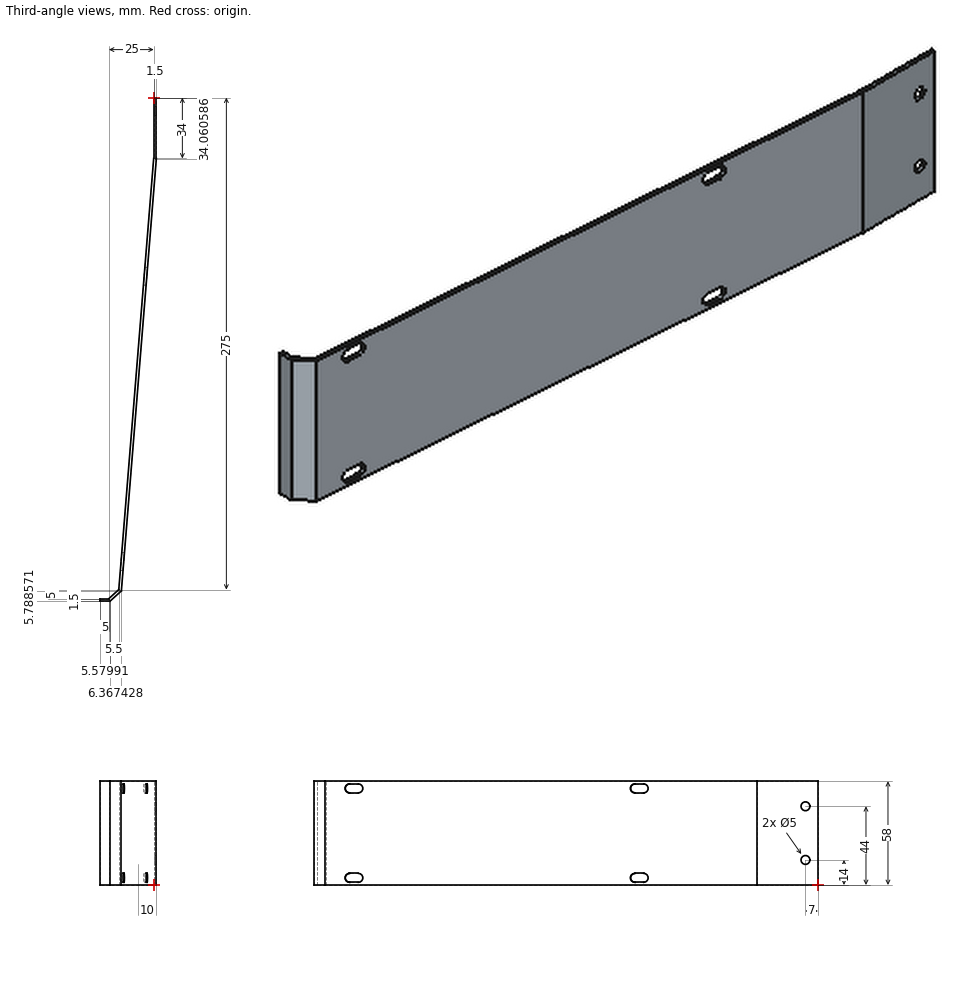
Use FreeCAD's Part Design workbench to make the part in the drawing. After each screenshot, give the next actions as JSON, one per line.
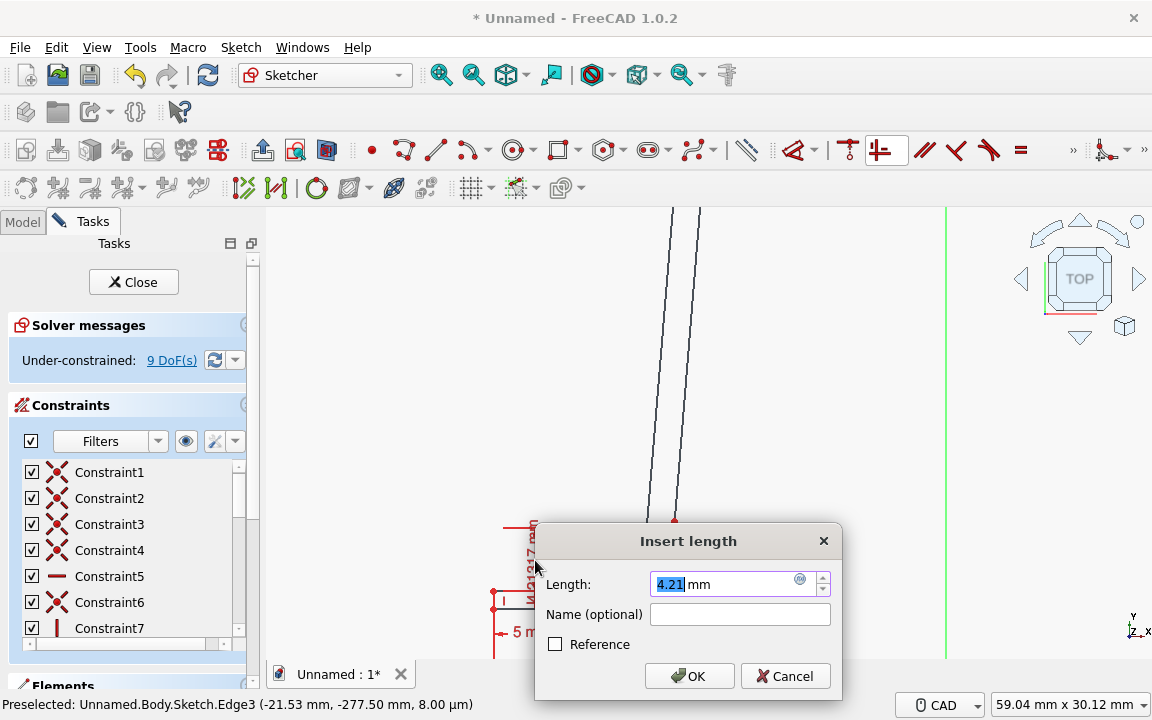
{"action": "type", "text": "5"}
{"action": "key", "text": "Return"}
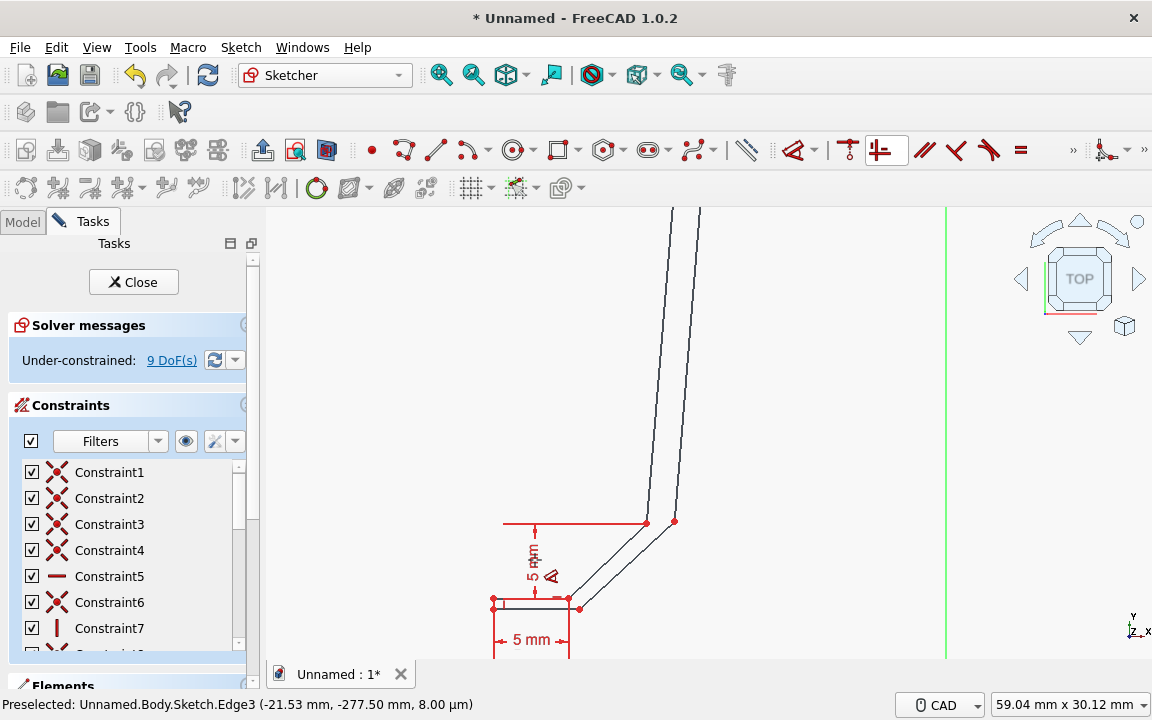
{"action": "scroll", "coordinate": [494, 604], "scroll_direction": "up", "scroll_amount": 3}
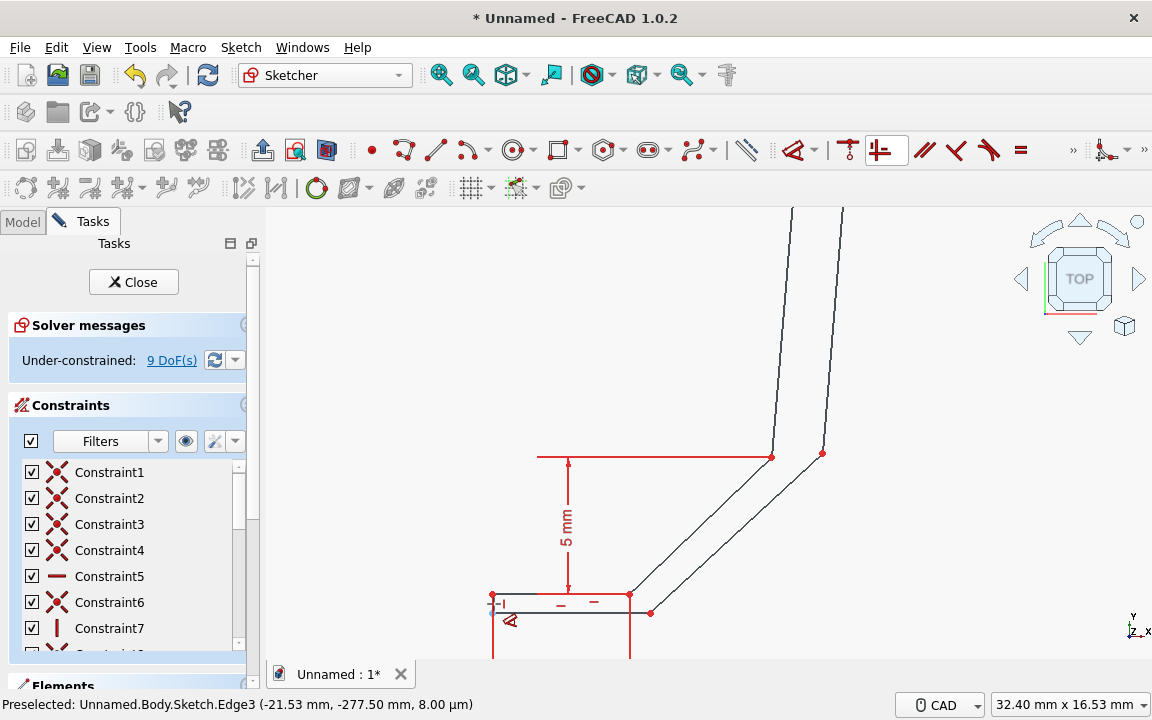
{"action": "left_click", "coordinate": [493, 604]}
{"action": "left_click", "coordinate": [459, 604]}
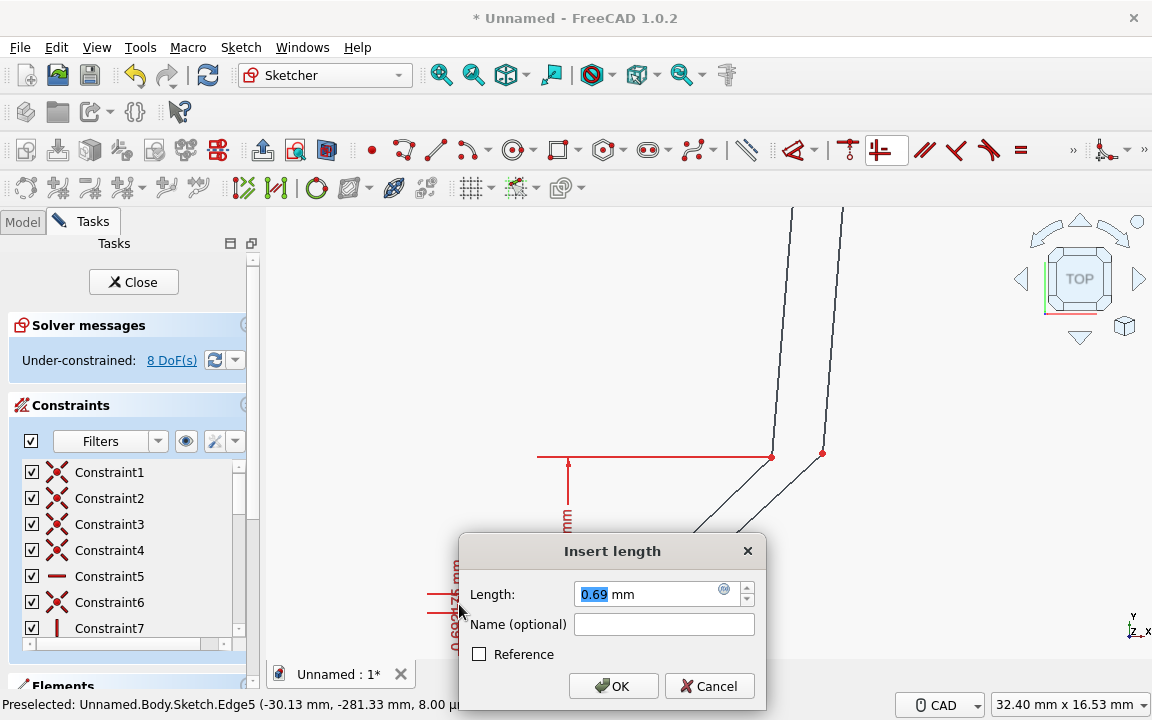
{"action": "type", "text": "1.5"}
{"action": "key", "text": "Return"}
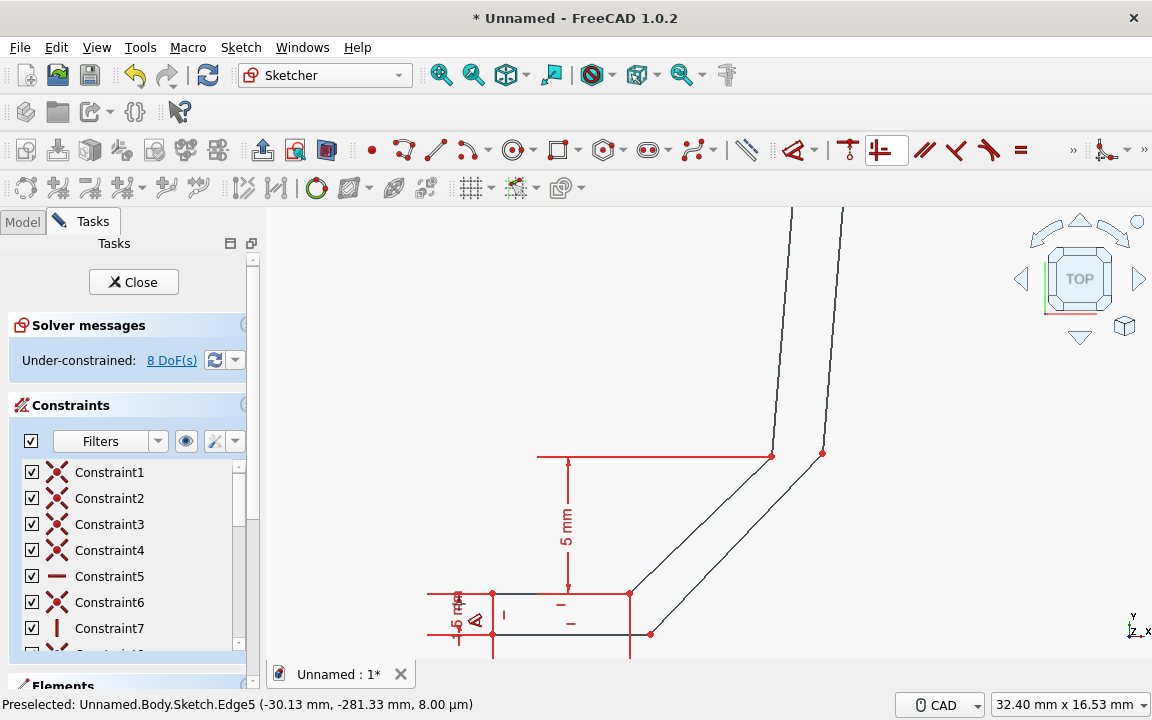
{"action": "scroll", "coordinate": [628, 589], "scroll_direction": "down", "scroll_amount": 16}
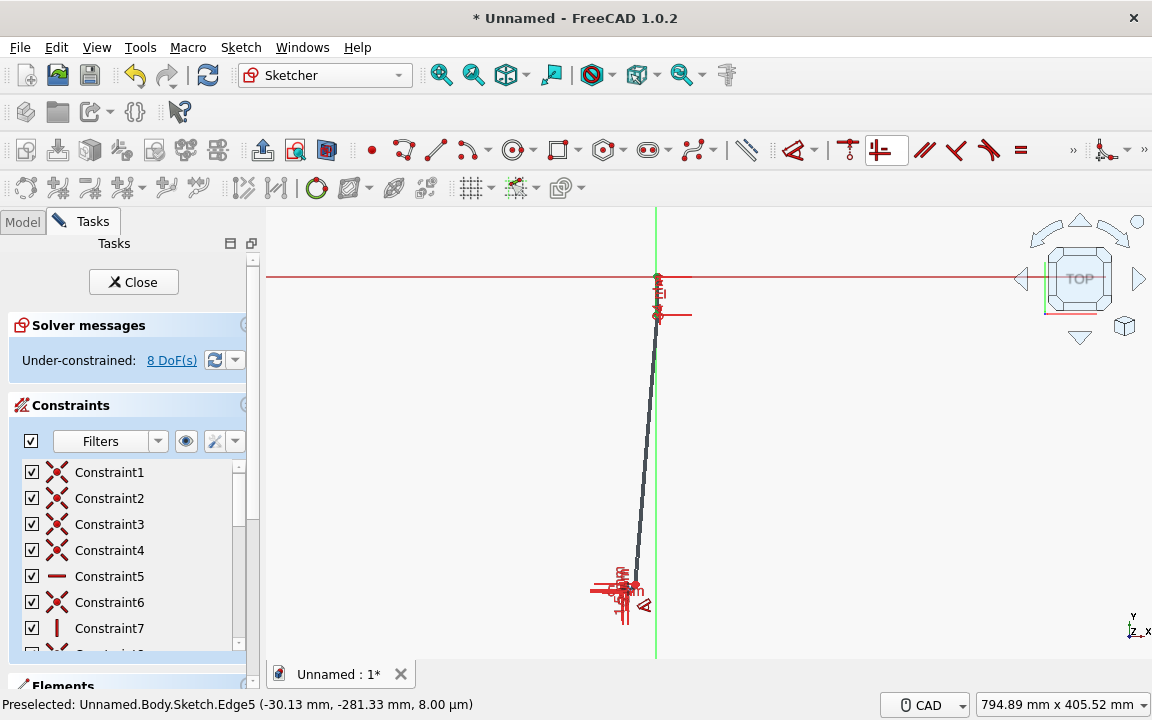
{"action": "scroll", "coordinate": [658, 277], "scroll_direction": "up", "scroll_amount": 16}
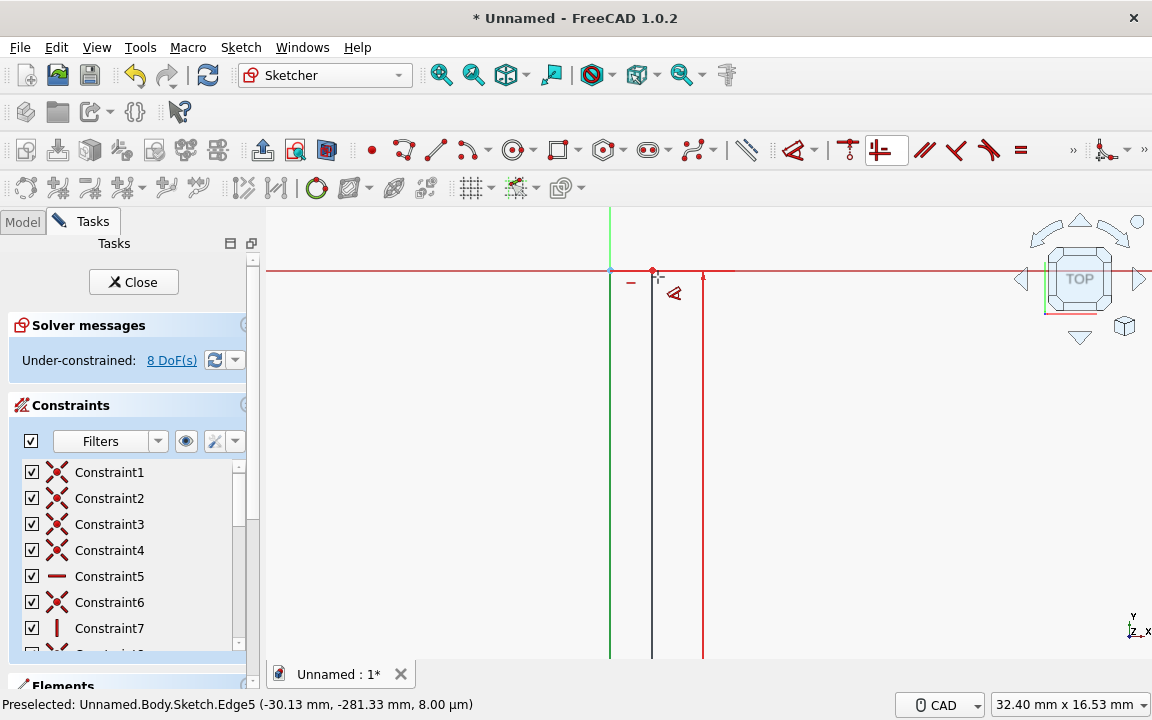
{"action": "left_click", "coordinate": [639, 271]}
{"action": "left_click", "coordinate": [631, 237]}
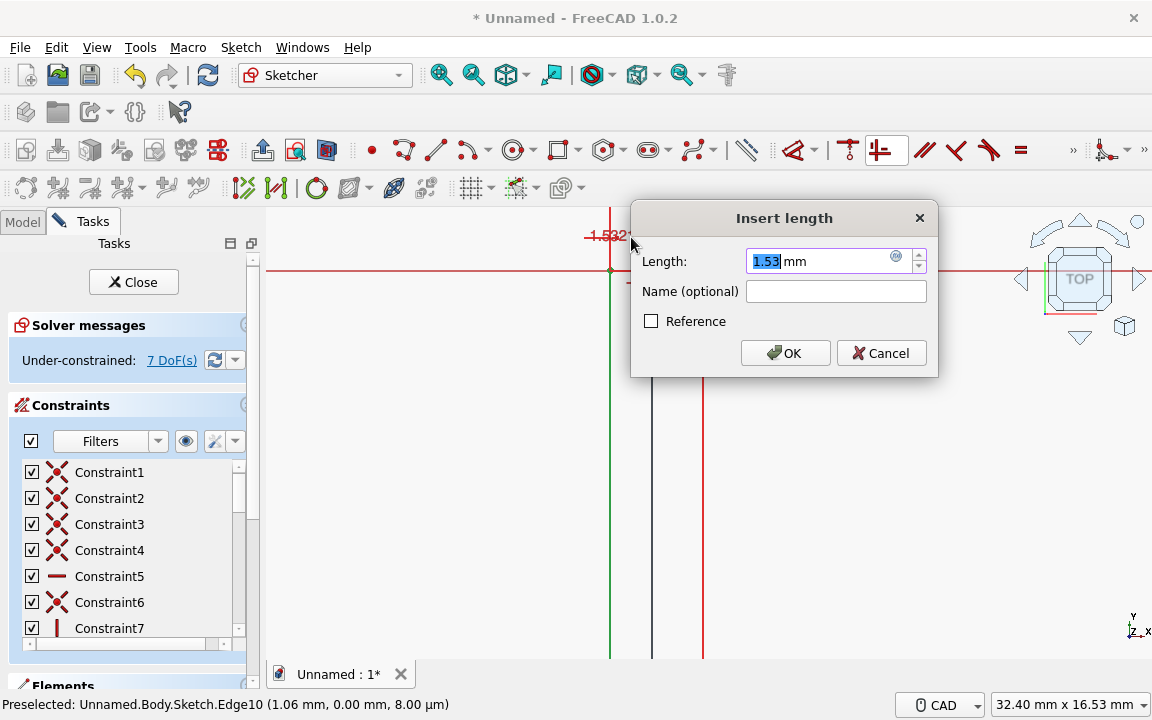
{"action": "type", "text": "1.5"}
{"action": "key", "text": "Return"}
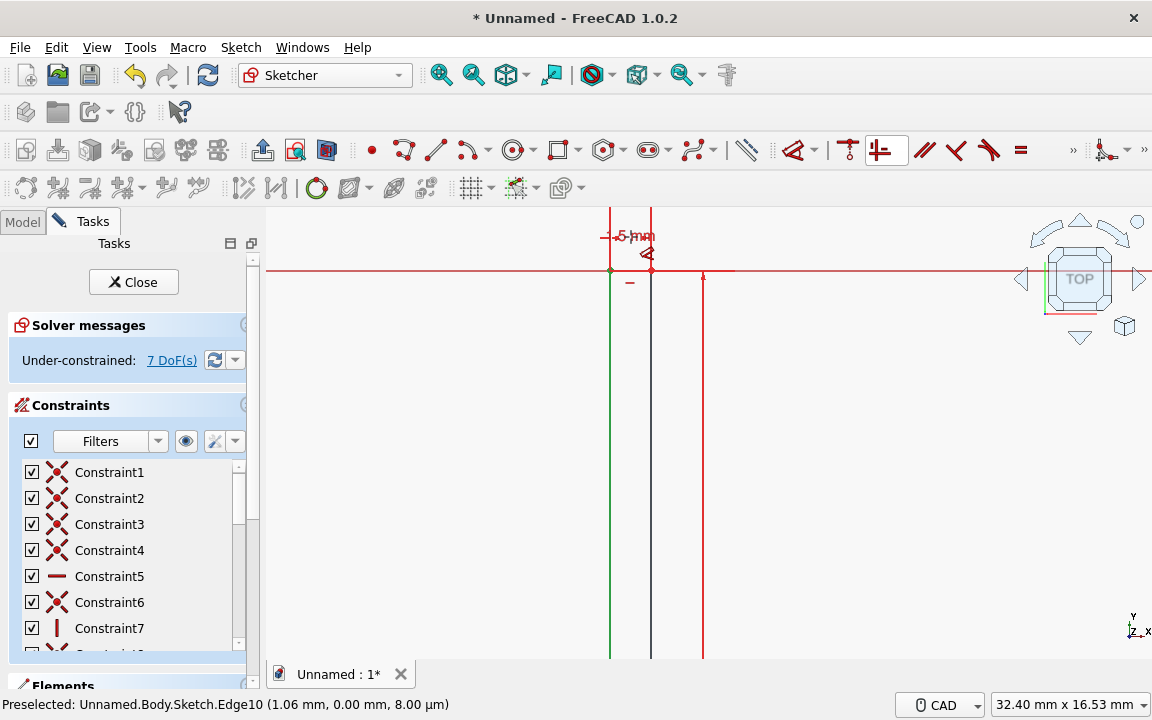
{"action": "scroll", "coordinate": [658, 276], "scroll_direction": "down", "scroll_amount": 16}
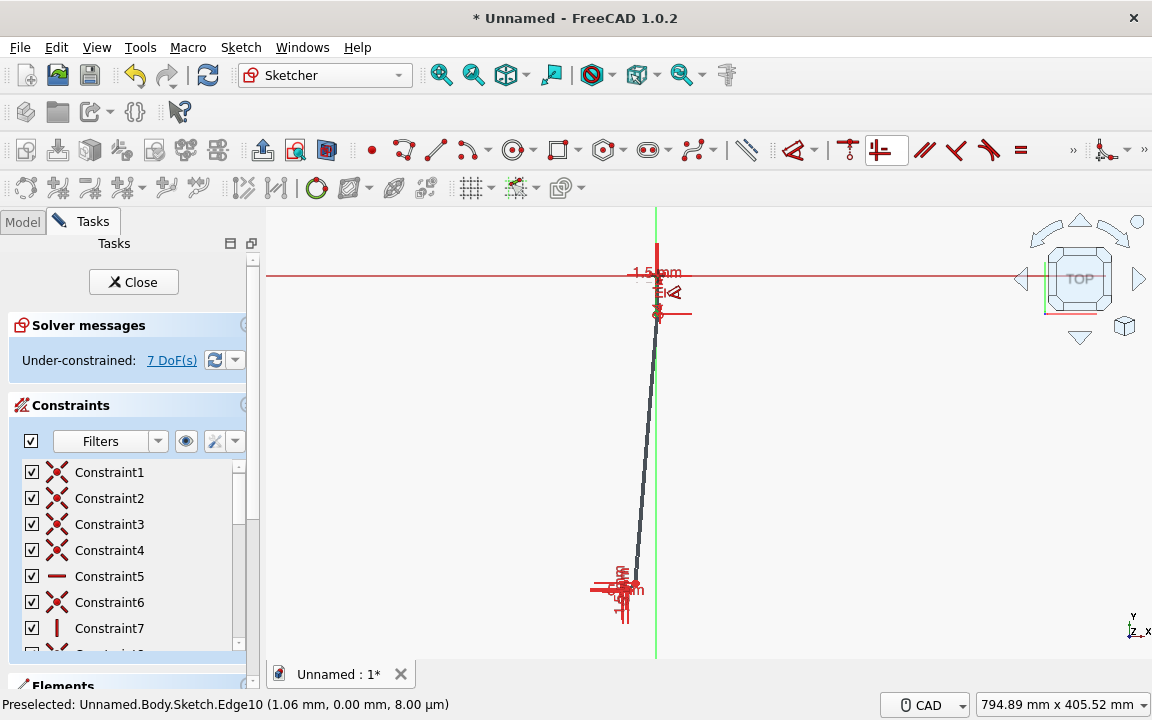
{"action": "scroll", "coordinate": [628, 589], "scroll_direction": "up", "scroll_amount": 10}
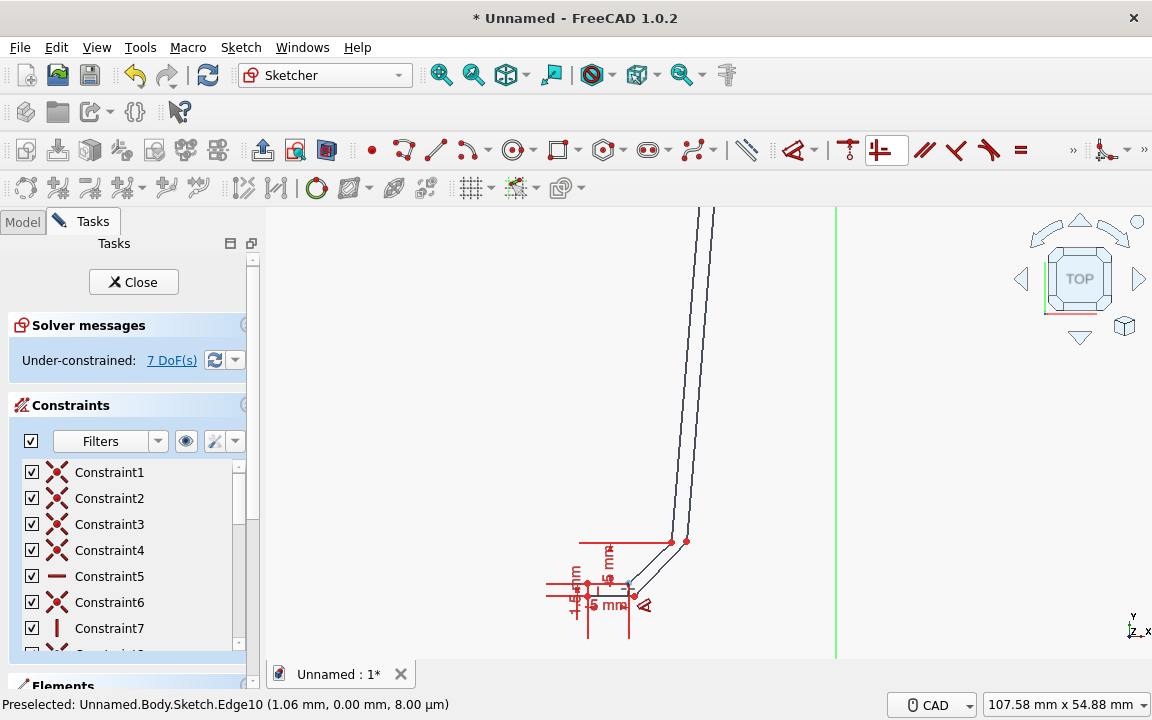
{"action": "left_click", "coordinate": [629, 584]}
{"action": "left_click", "coordinate": [732, 618]}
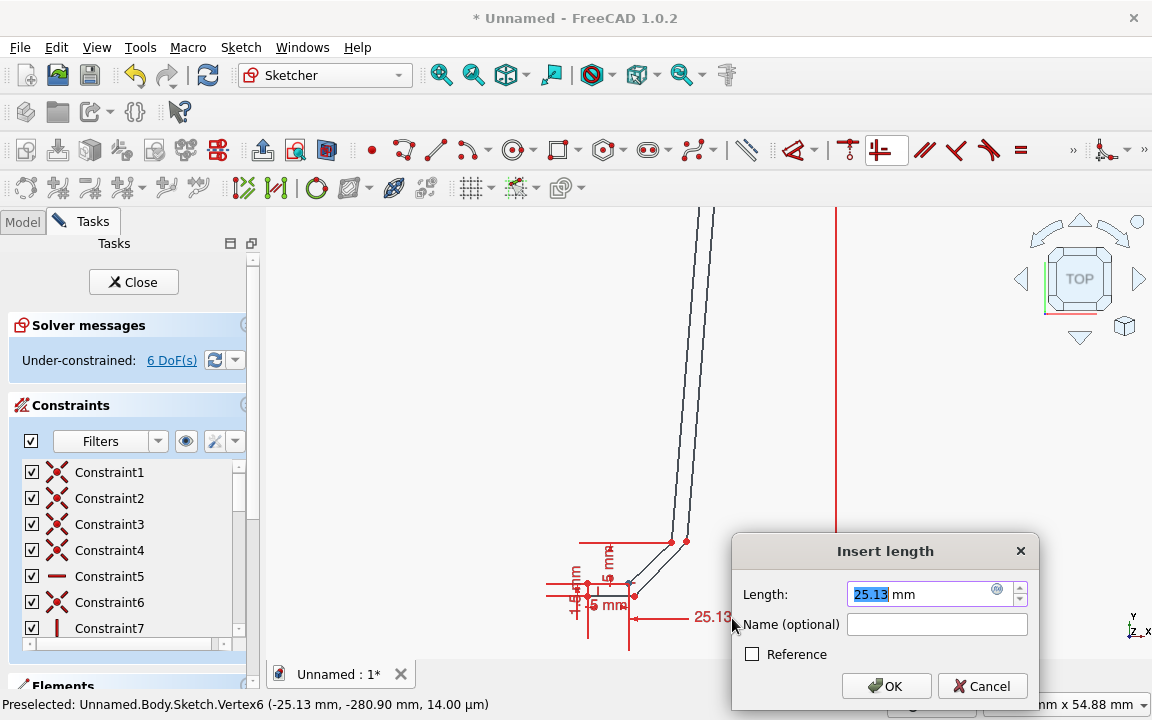
{"action": "type", "text": "25"}
{"action": "key", "text": "Return"}